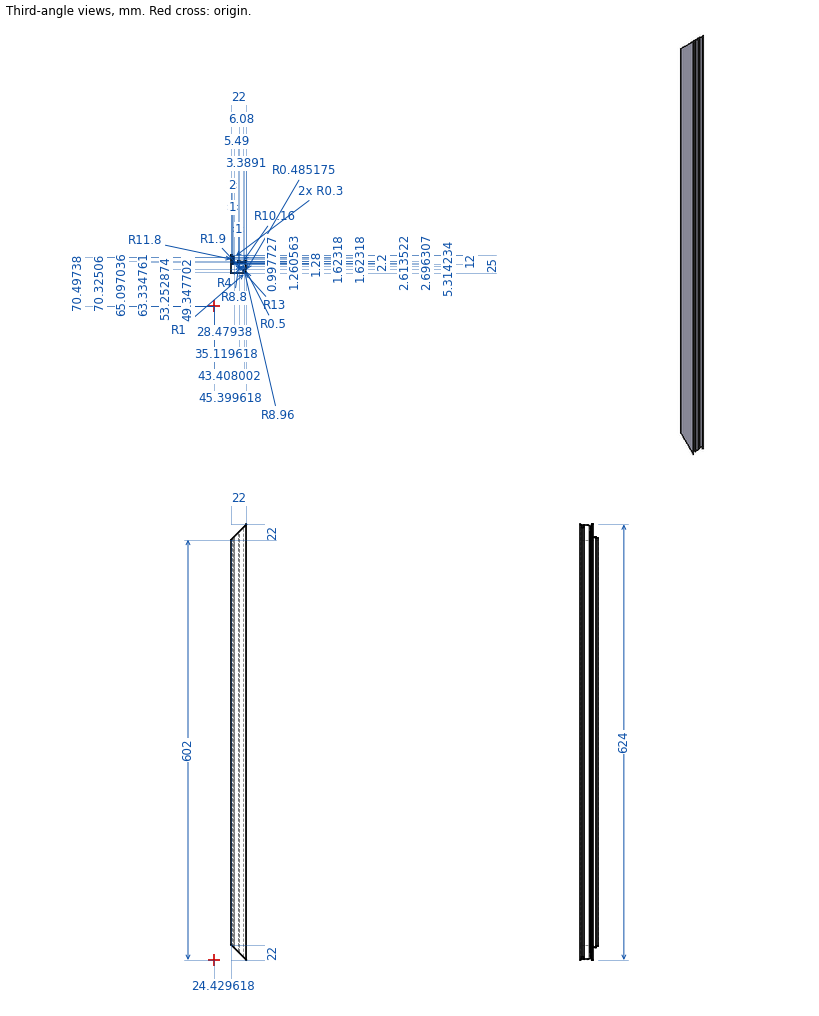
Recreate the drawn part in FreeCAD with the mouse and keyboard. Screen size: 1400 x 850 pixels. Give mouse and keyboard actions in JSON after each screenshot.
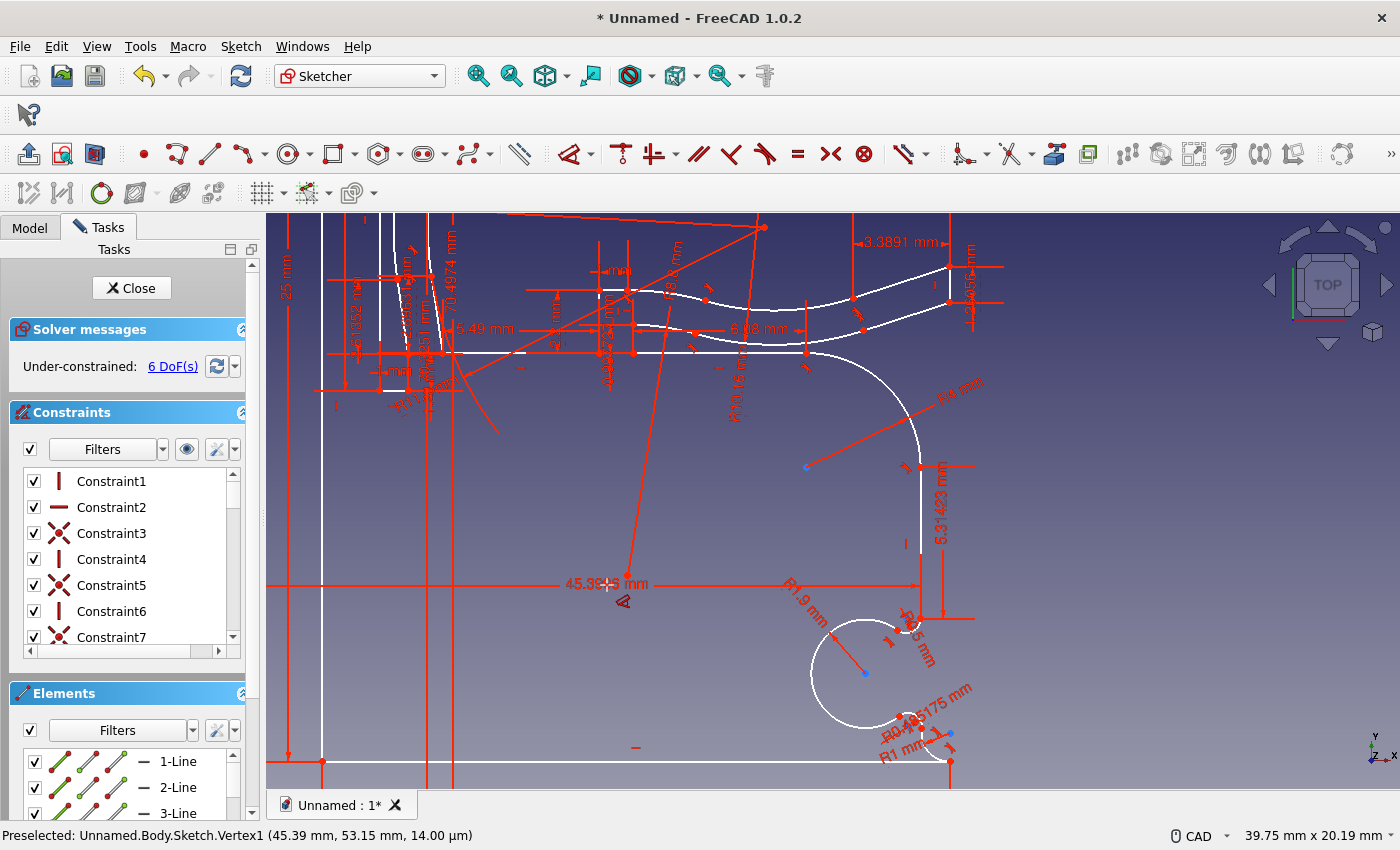
{"action": "left_click", "coordinate": [921, 619]}
{"action": "left_click", "coordinate": [955, 690]}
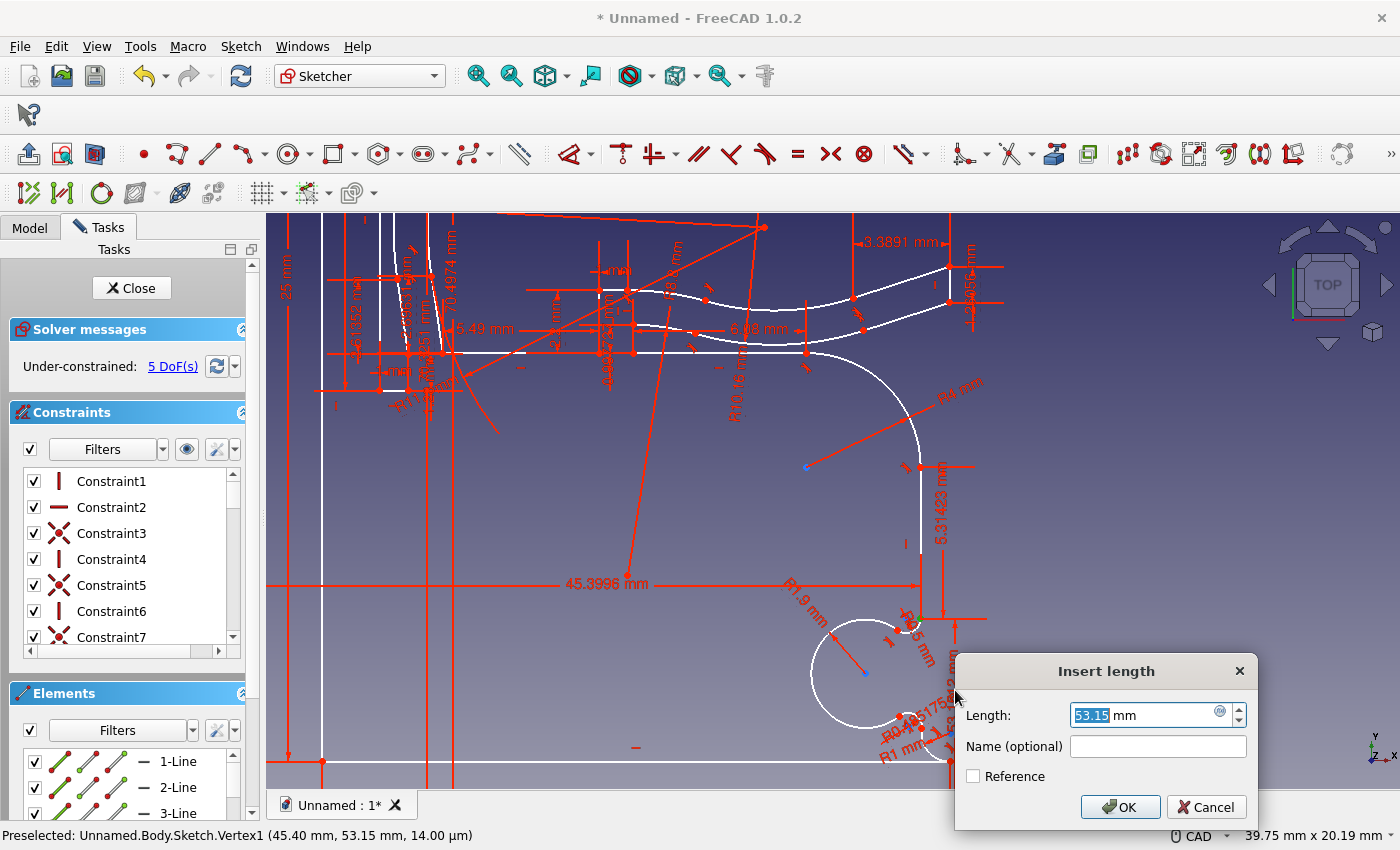
{"action": "type", "text": "53.252874"}
{"action": "key", "text": "Return"}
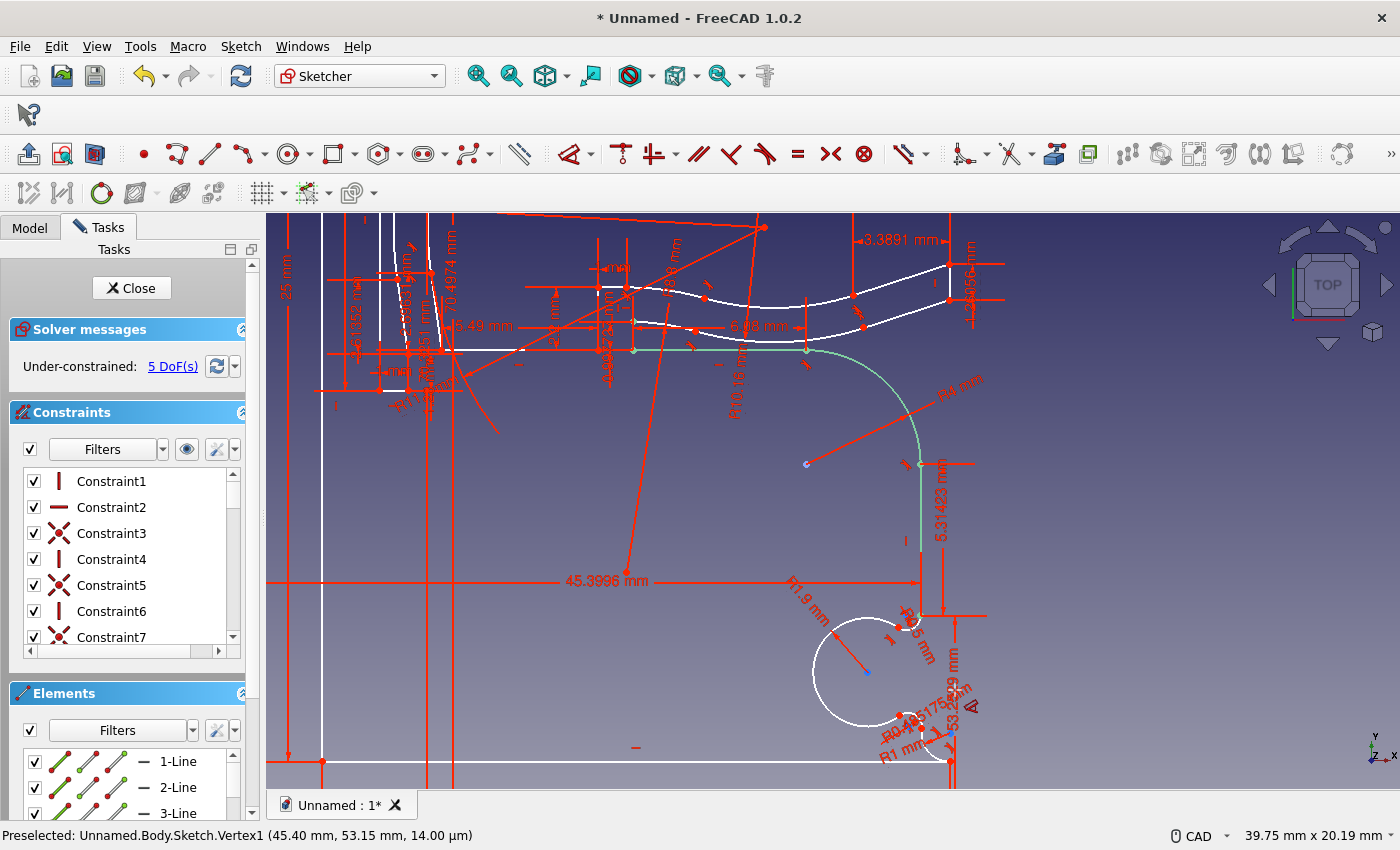
{"action": "left_click", "coordinate": [864, 328]}
{"action": "left_click", "coordinate": [579, 294]}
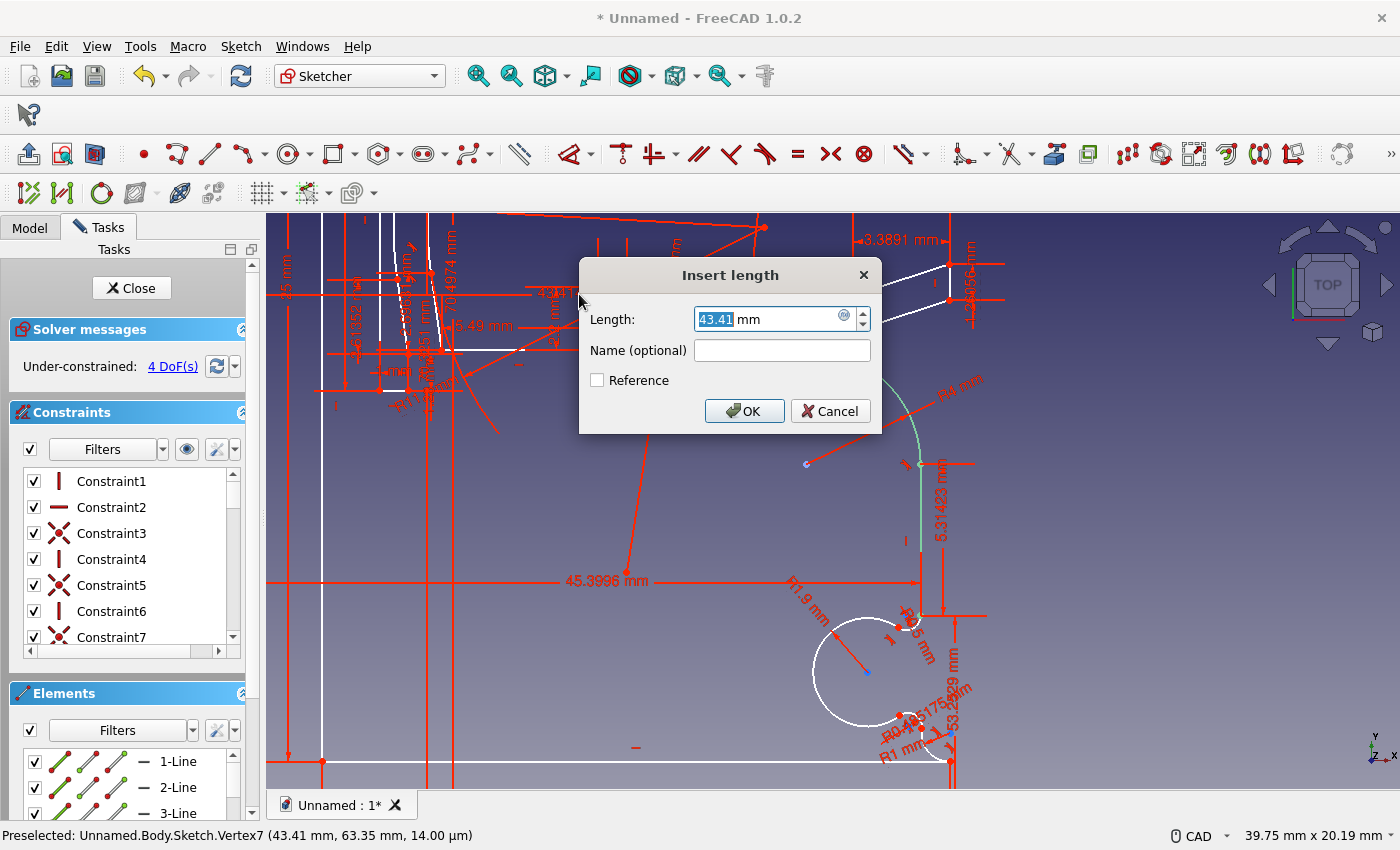
{"action": "type", "text": "43.408002"}
{"action": "key", "text": "Return"}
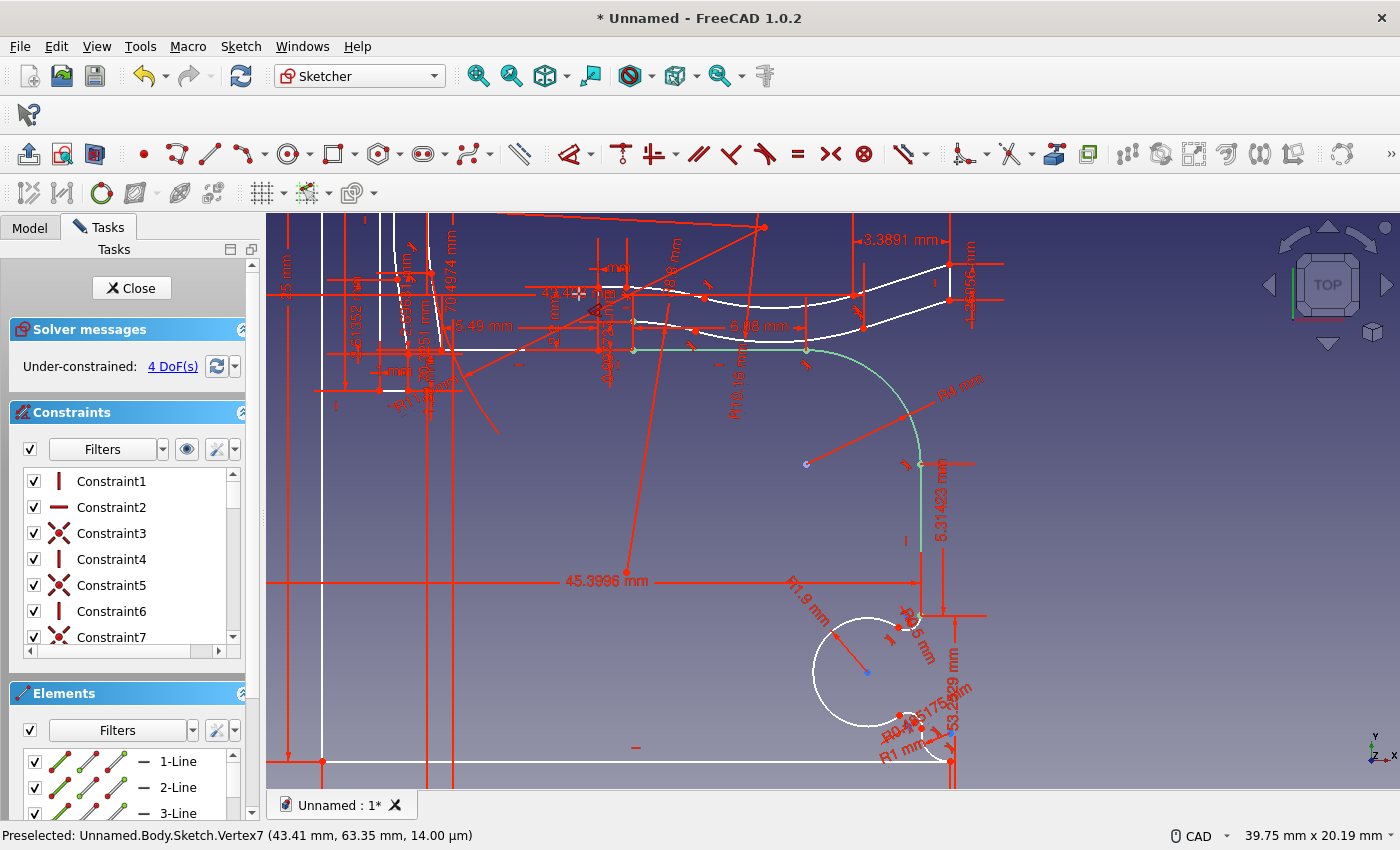
{"action": "left_click", "coordinate": [864, 328]}
{"action": "left_click", "coordinate": [898, 545]}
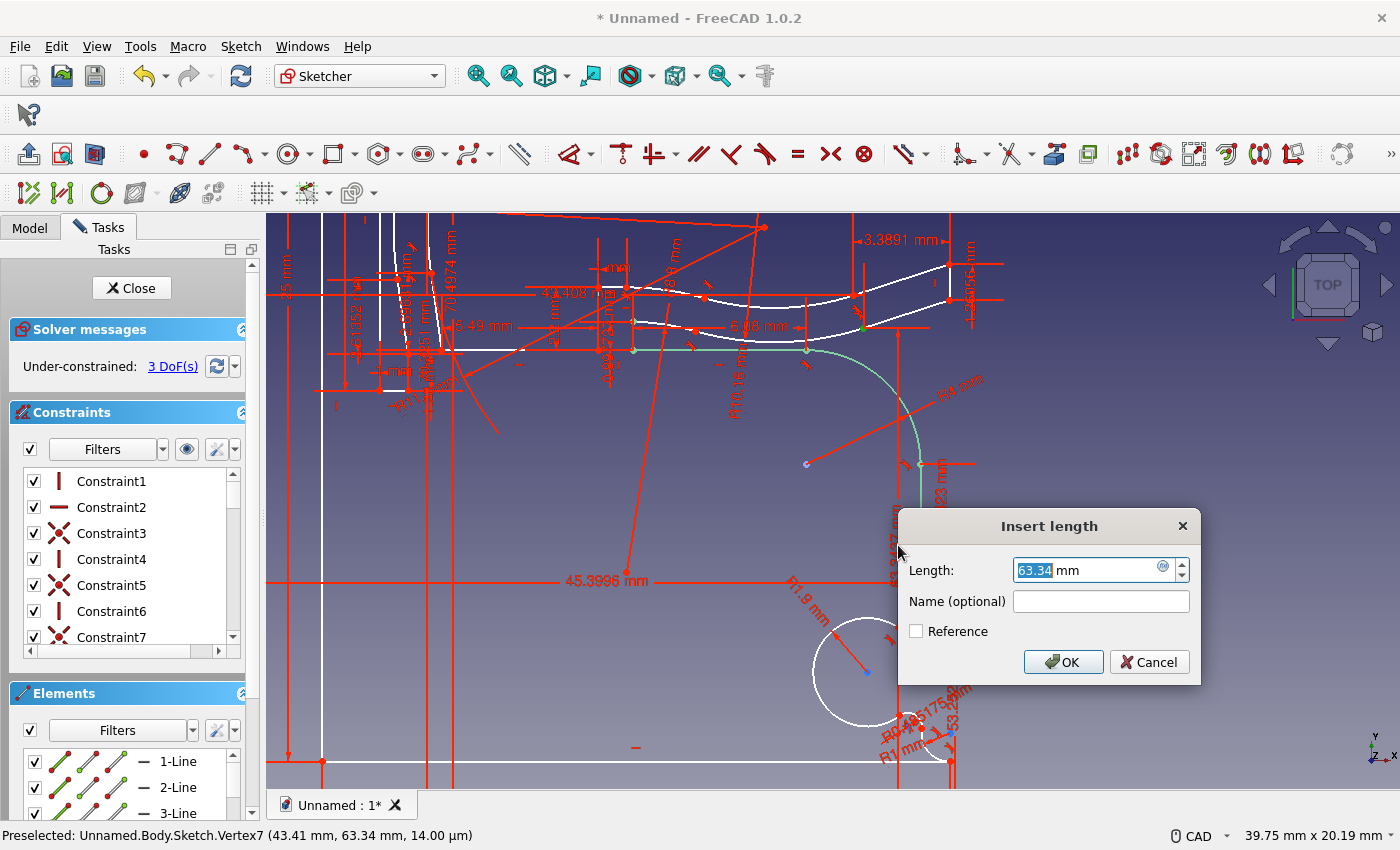
{"action": "type", "text": "63.334761"}
{"action": "key", "text": "Return"}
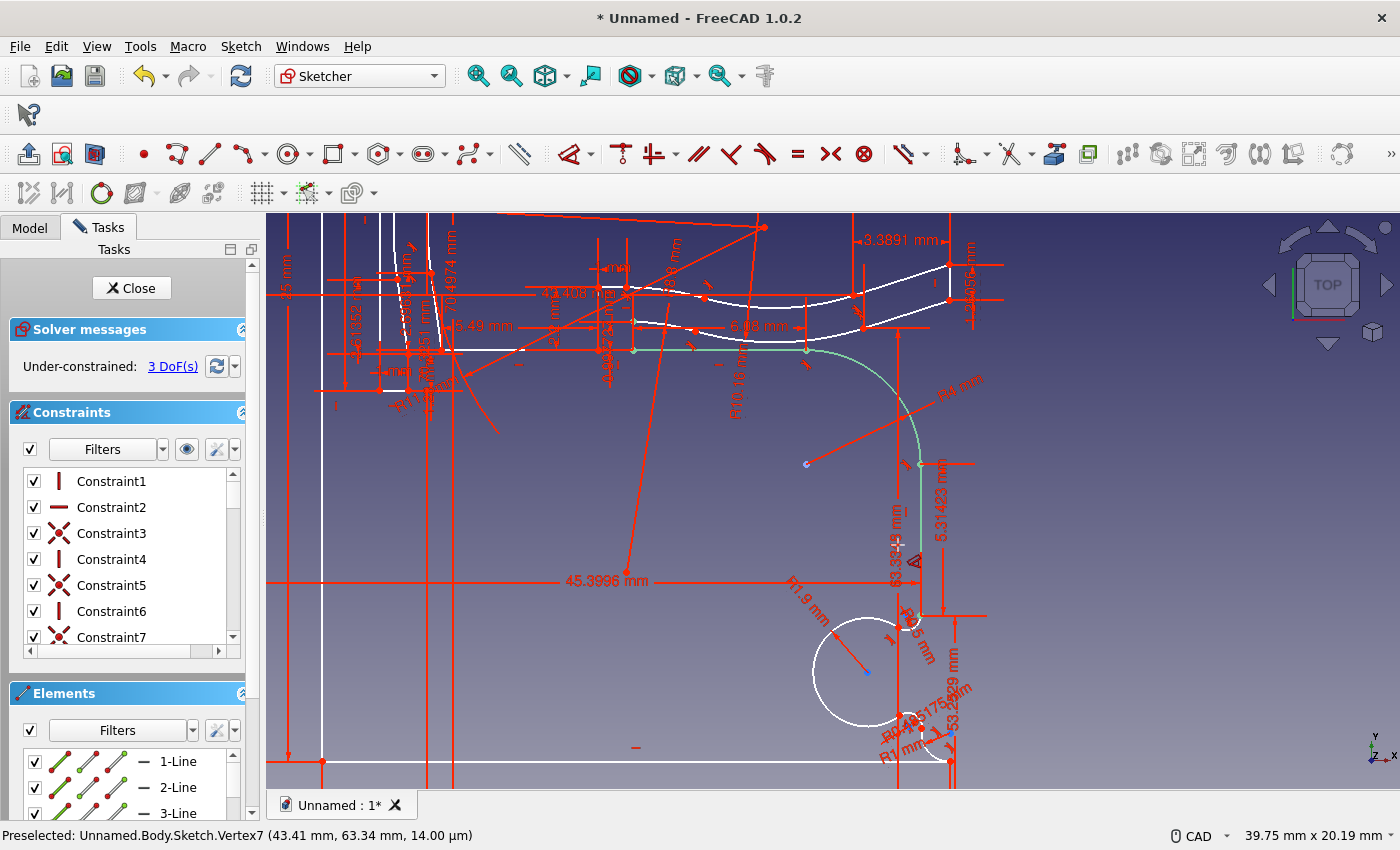
{"action": "left_click", "coordinate": [627, 287]}
{"action": "left_click", "coordinate": [537, 253]}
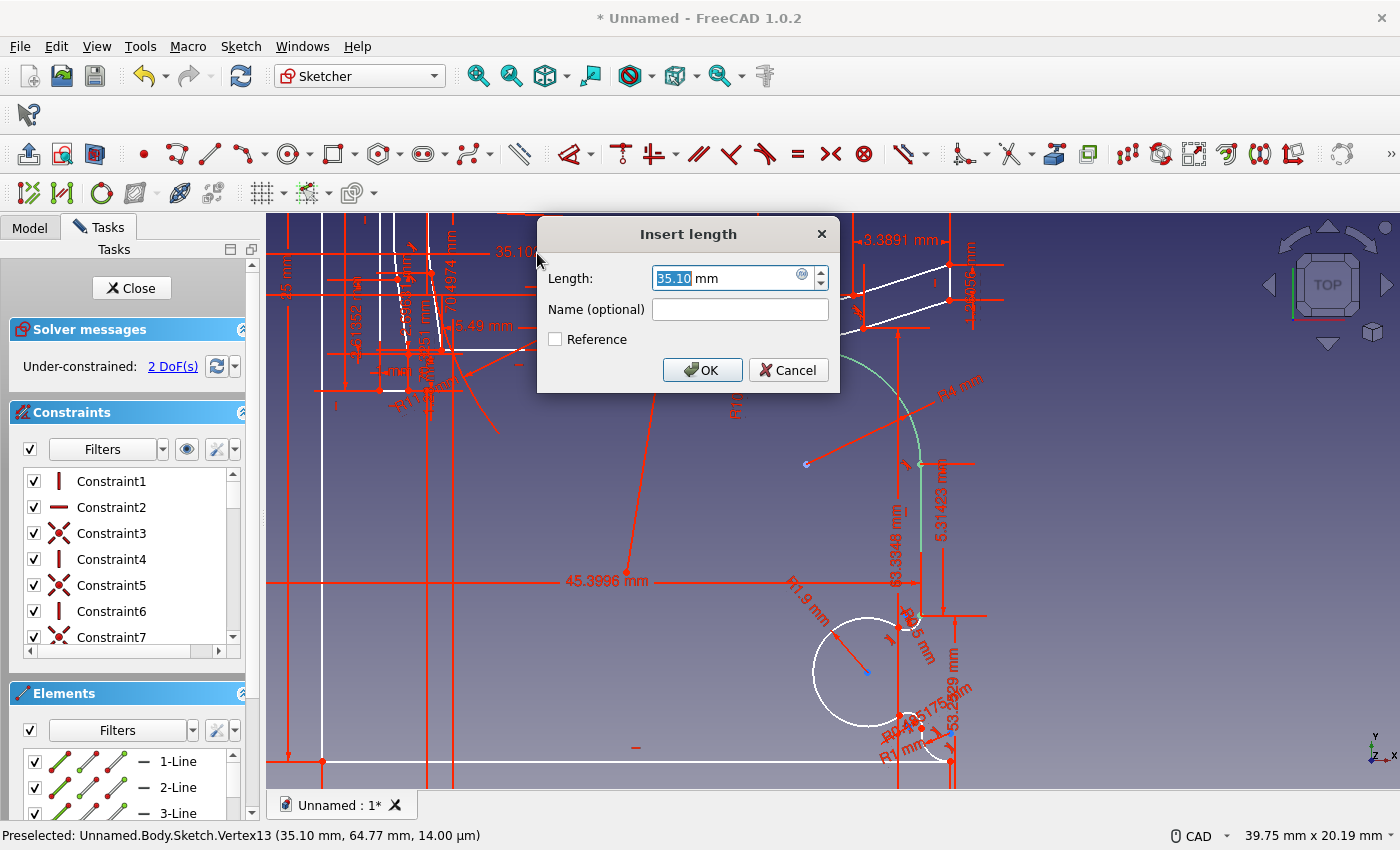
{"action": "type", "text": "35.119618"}
{"action": "key", "text": "Return"}